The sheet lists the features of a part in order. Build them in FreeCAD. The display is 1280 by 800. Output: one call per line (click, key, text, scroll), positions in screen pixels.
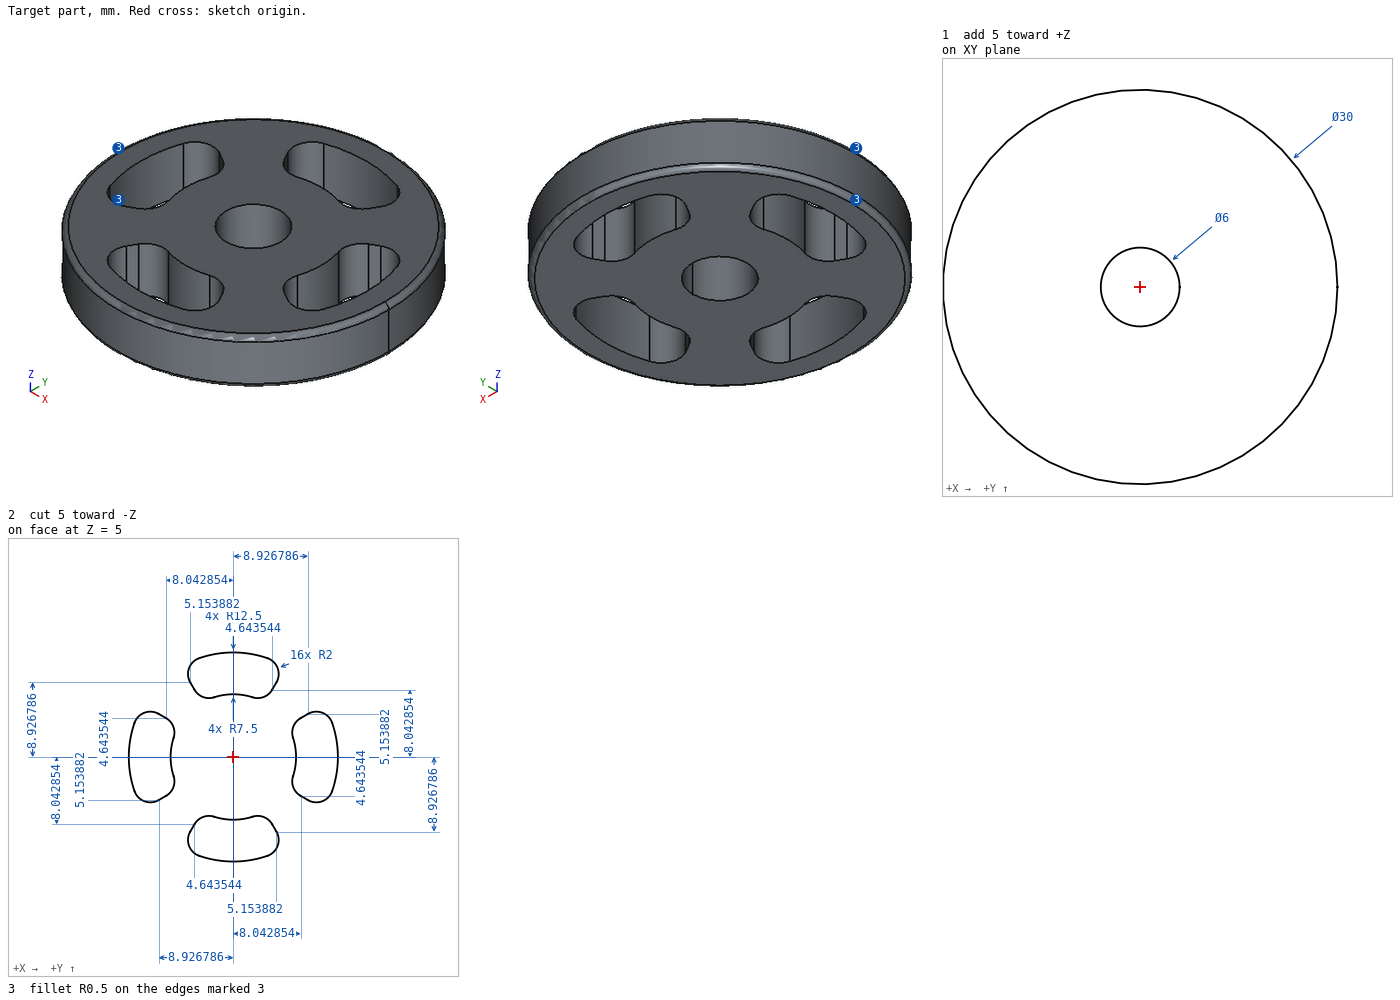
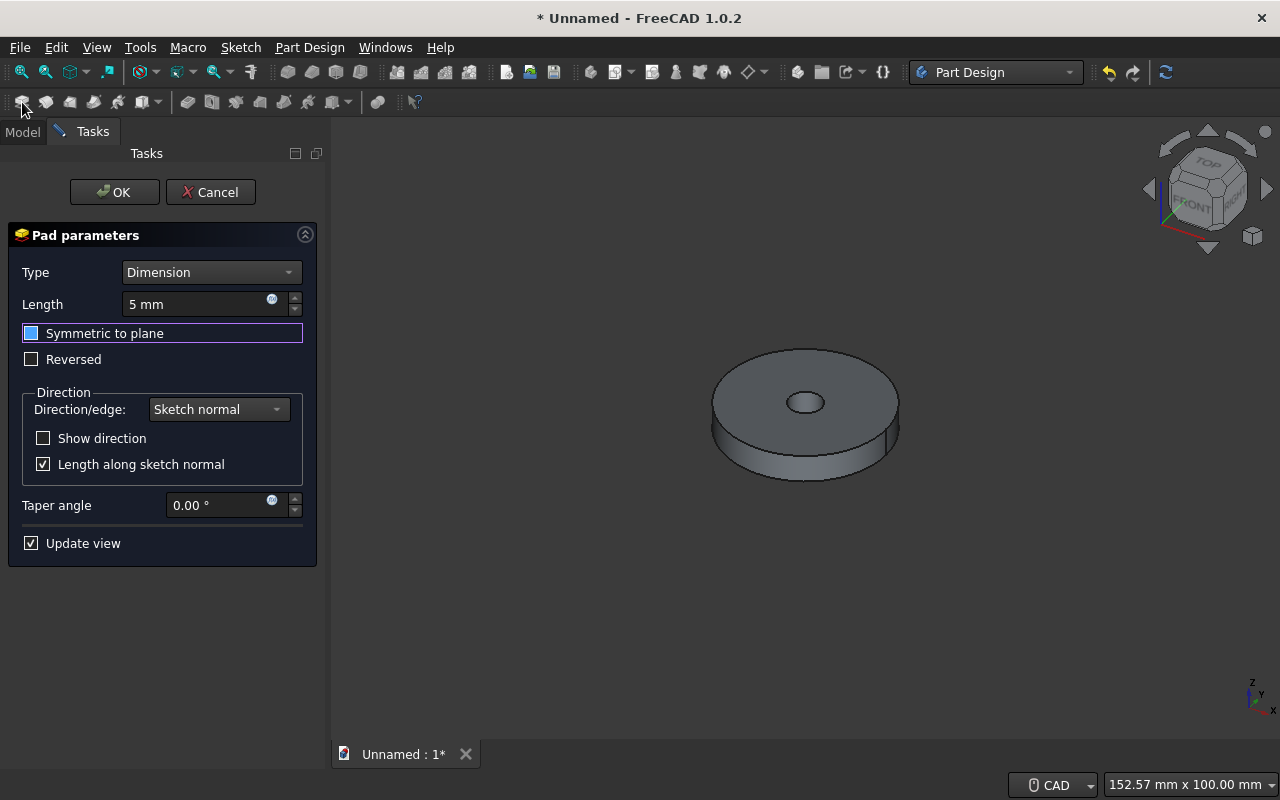
click(115, 192)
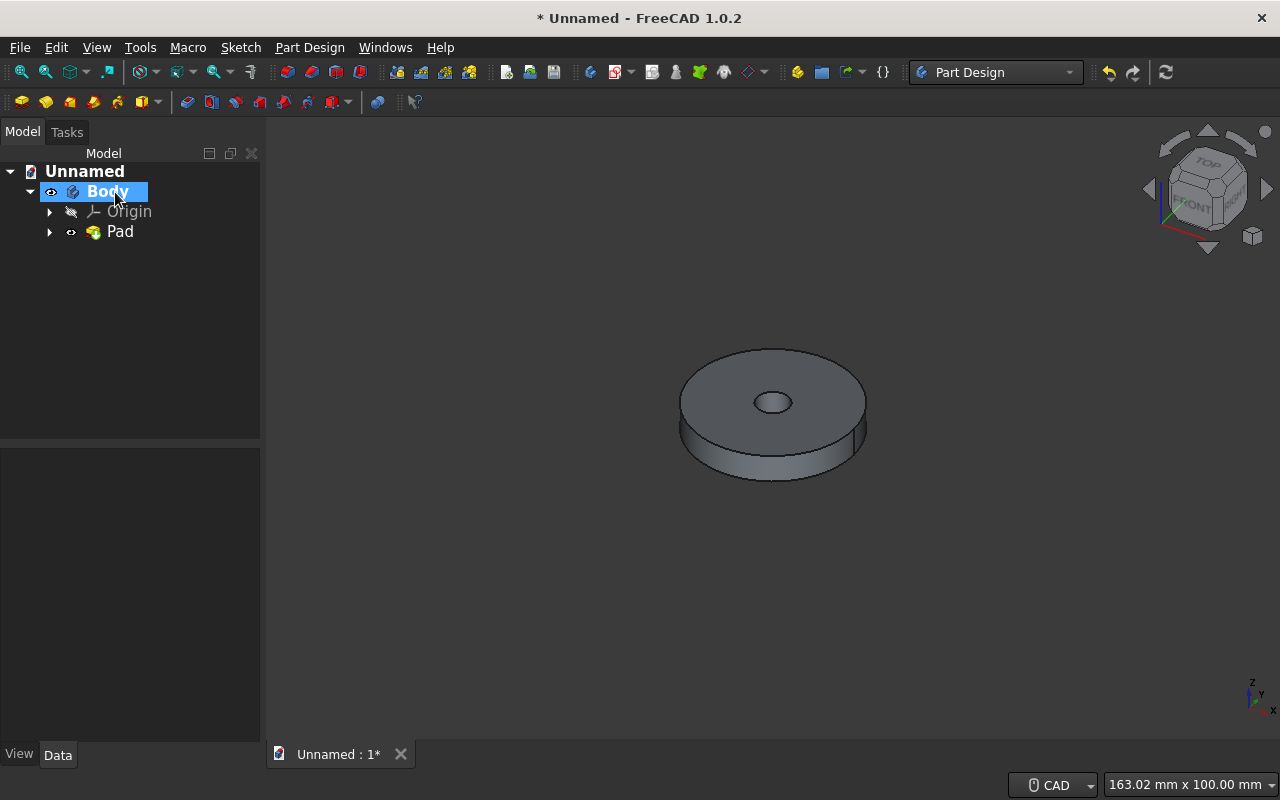
click(22, 72)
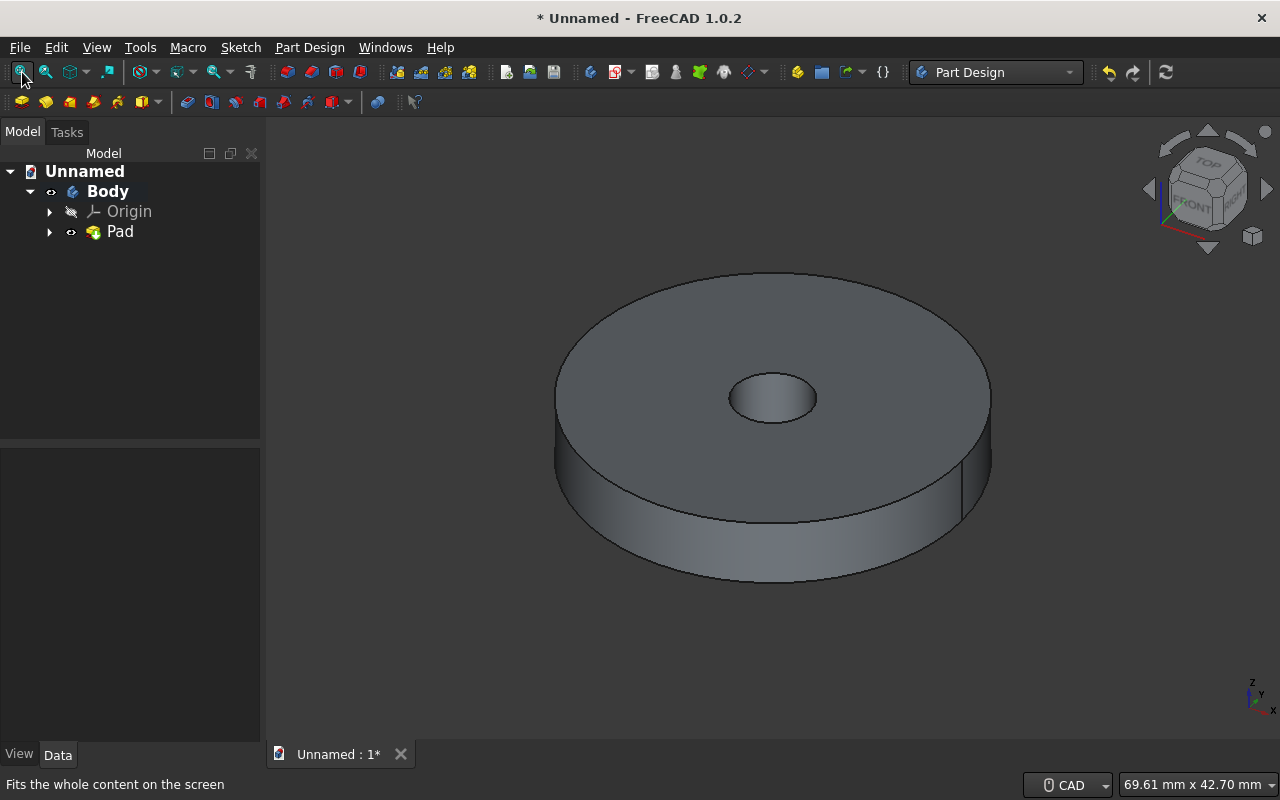
click(881, 433)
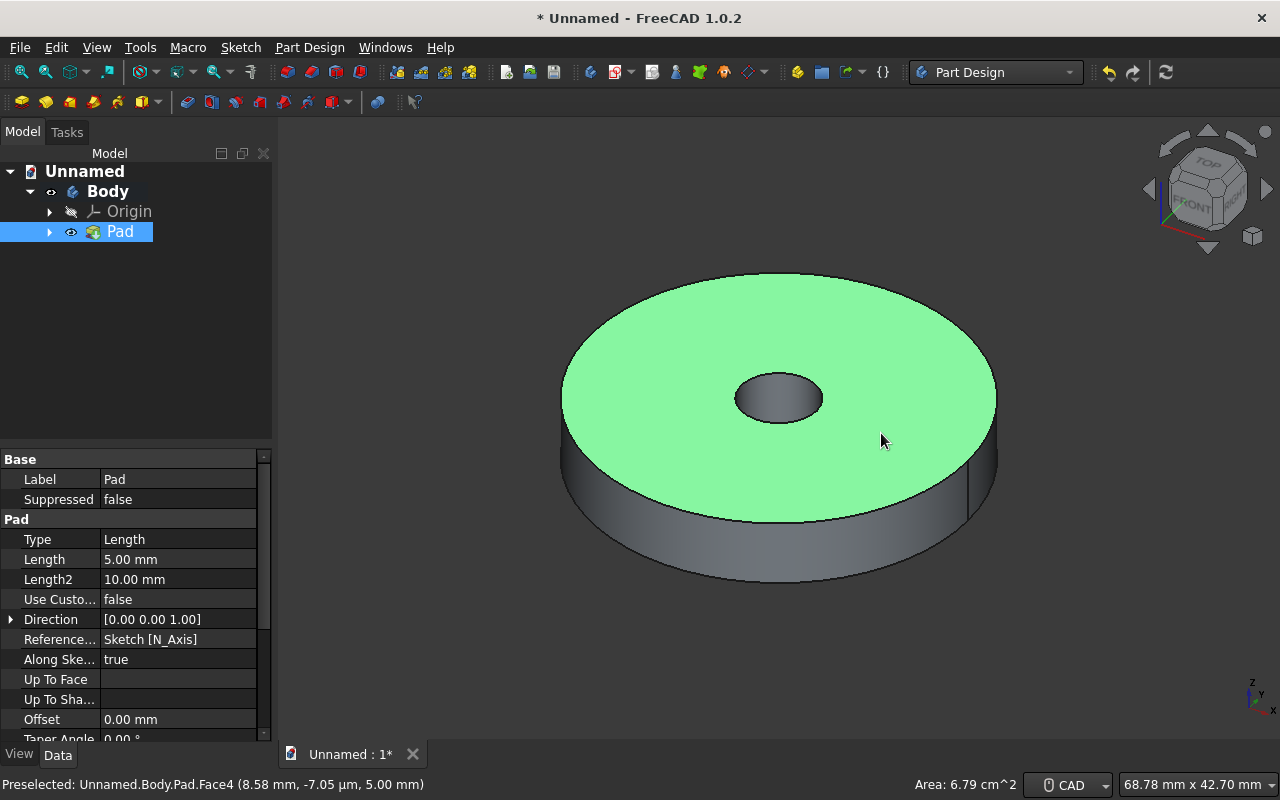
click(616, 72)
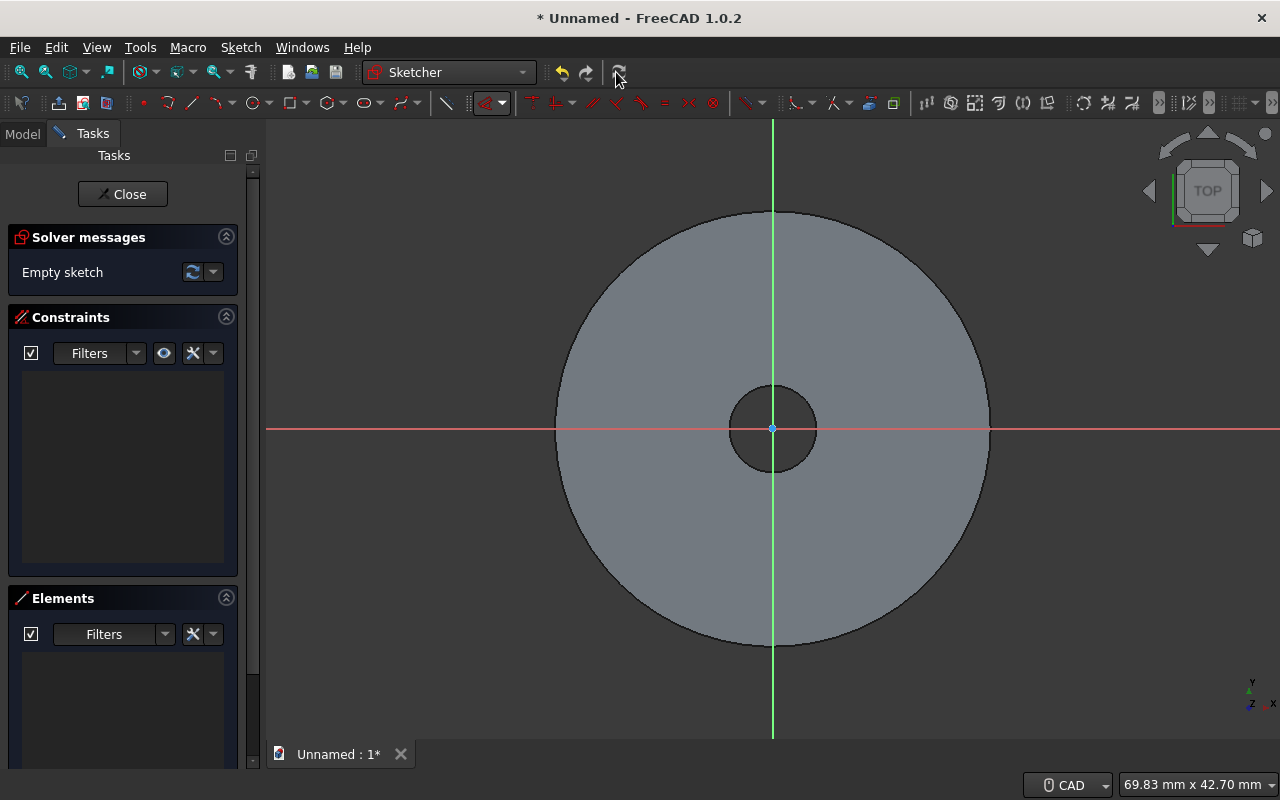
click(192, 104)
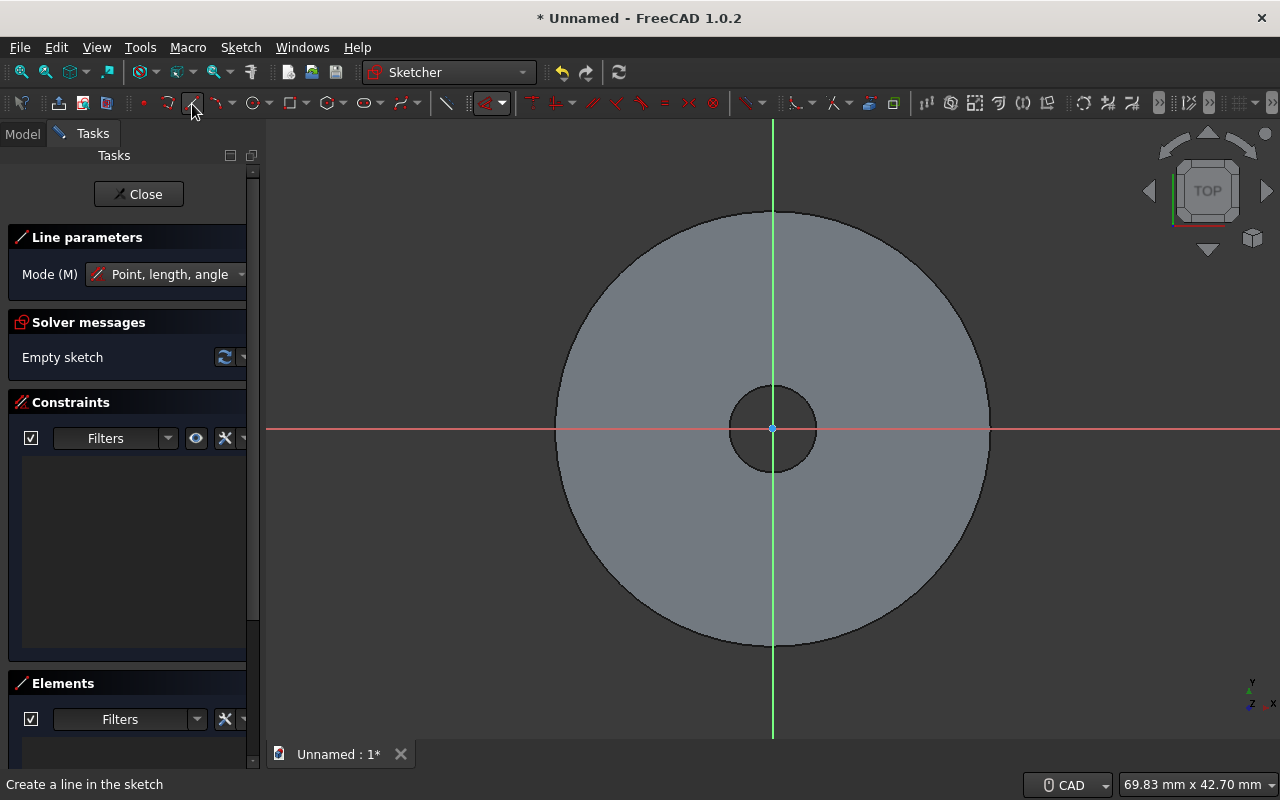
click(698, 299)
click(705, 312)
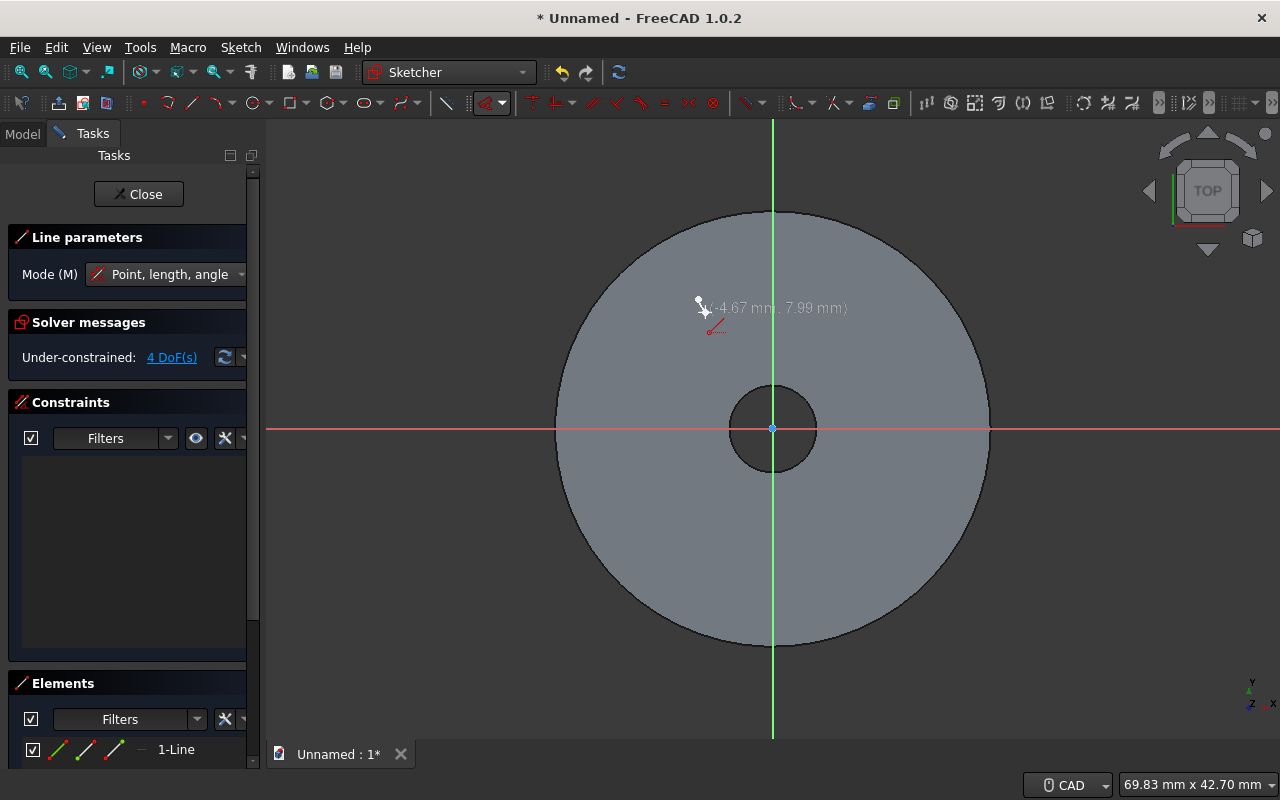
click(840, 312)
click(848, 299)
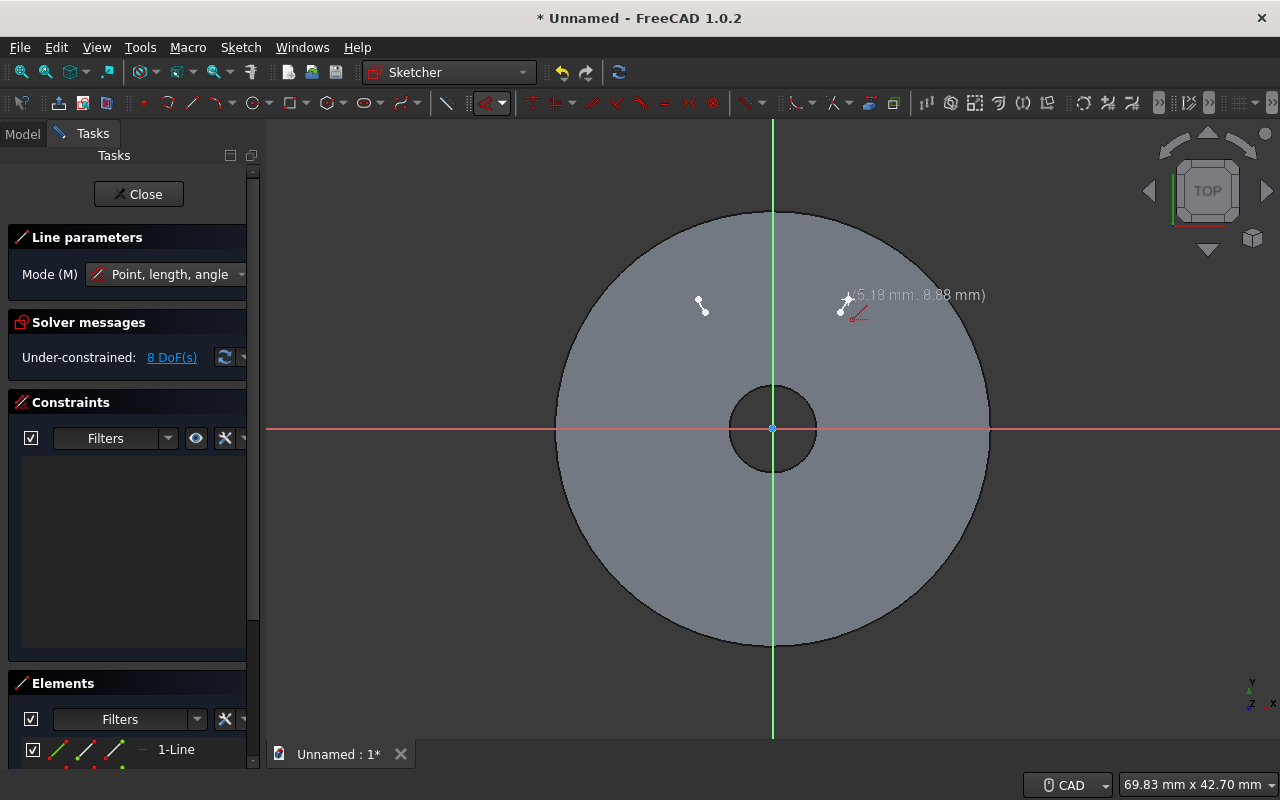
click(216, 104)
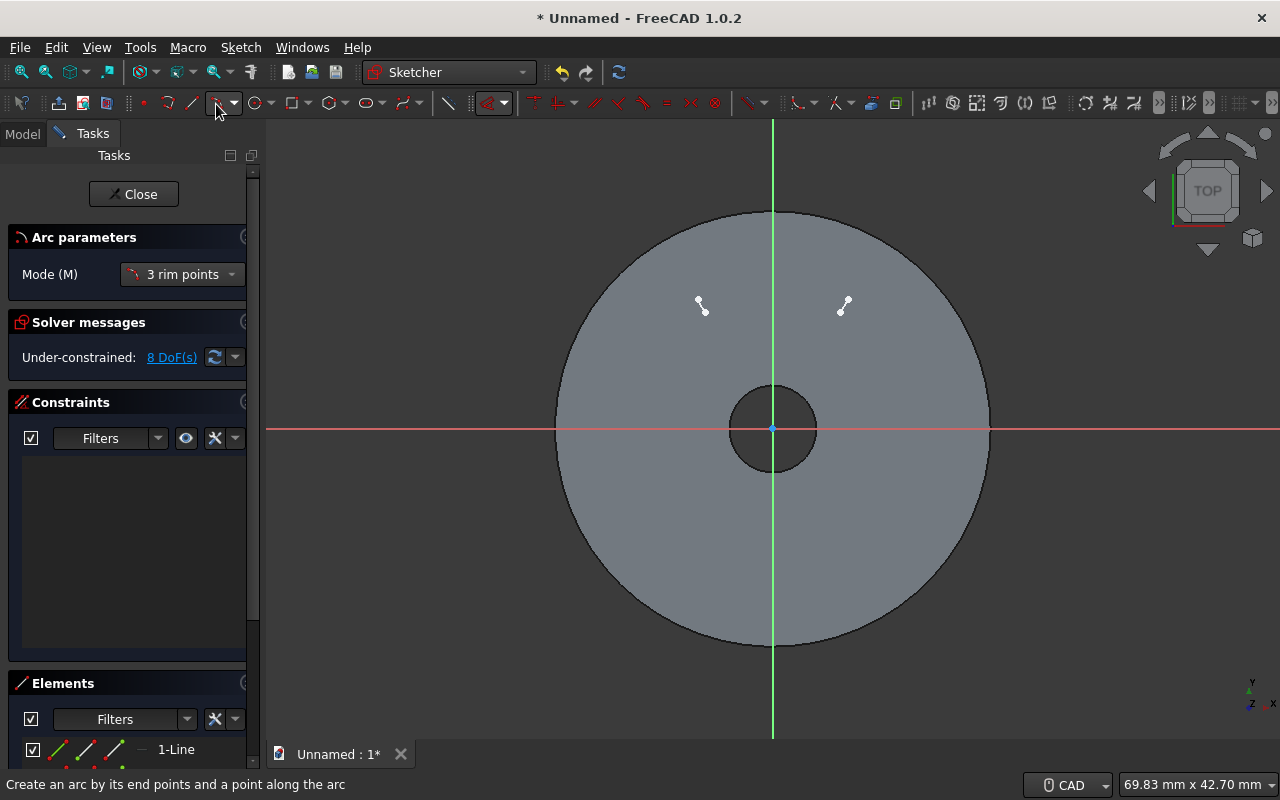
scroll(705, 312, up, 4)